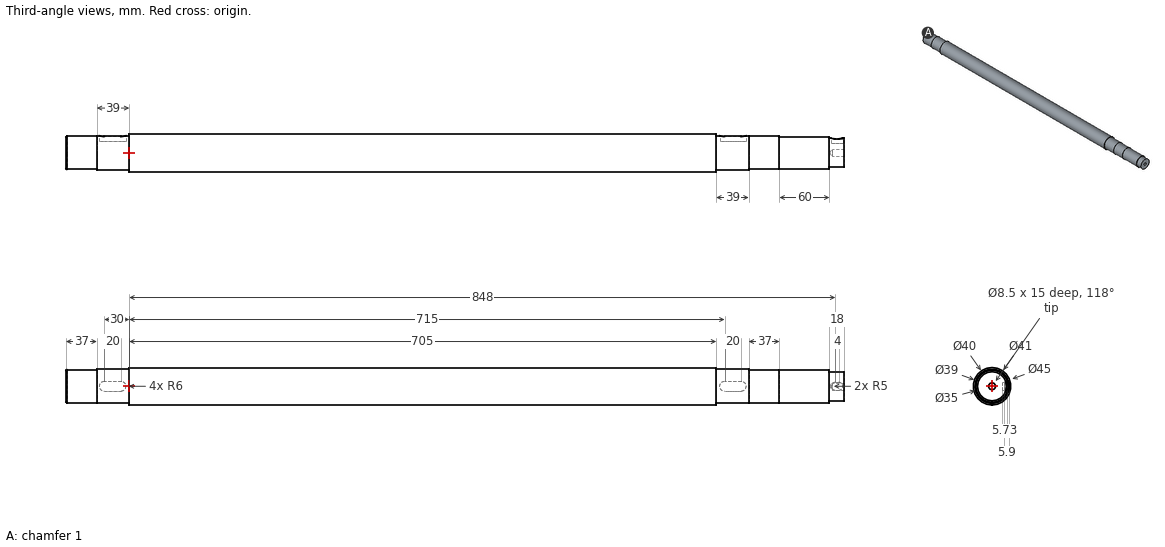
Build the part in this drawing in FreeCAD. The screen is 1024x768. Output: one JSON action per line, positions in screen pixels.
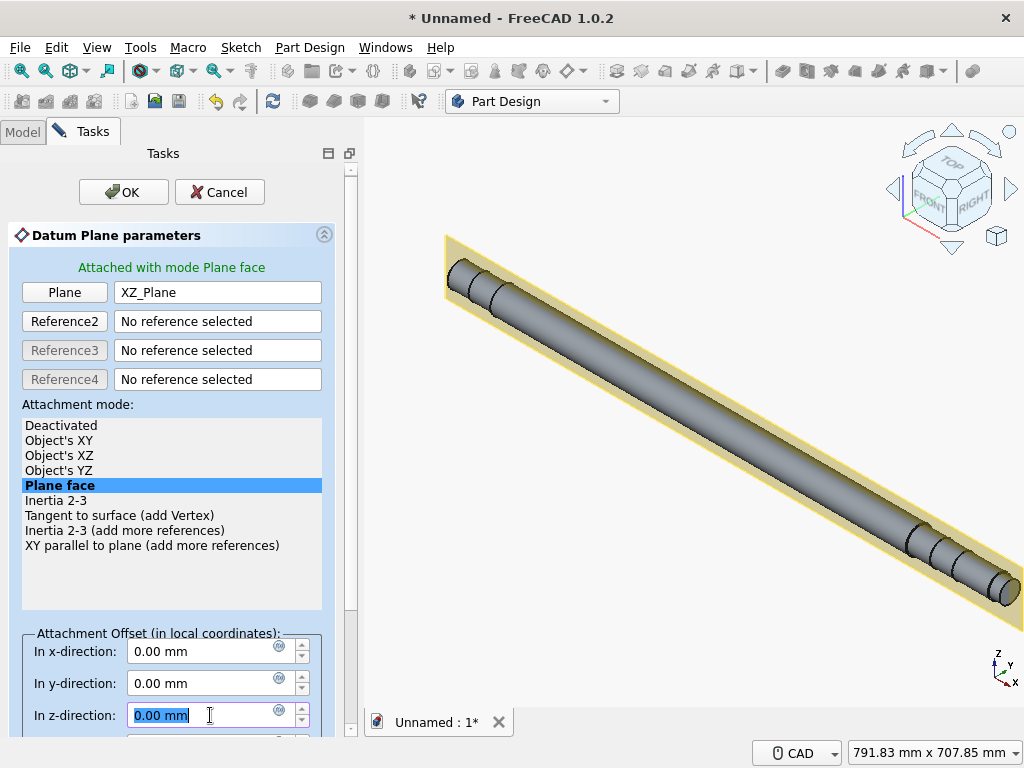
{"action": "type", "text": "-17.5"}
{"action": "key", "text": "Tab"}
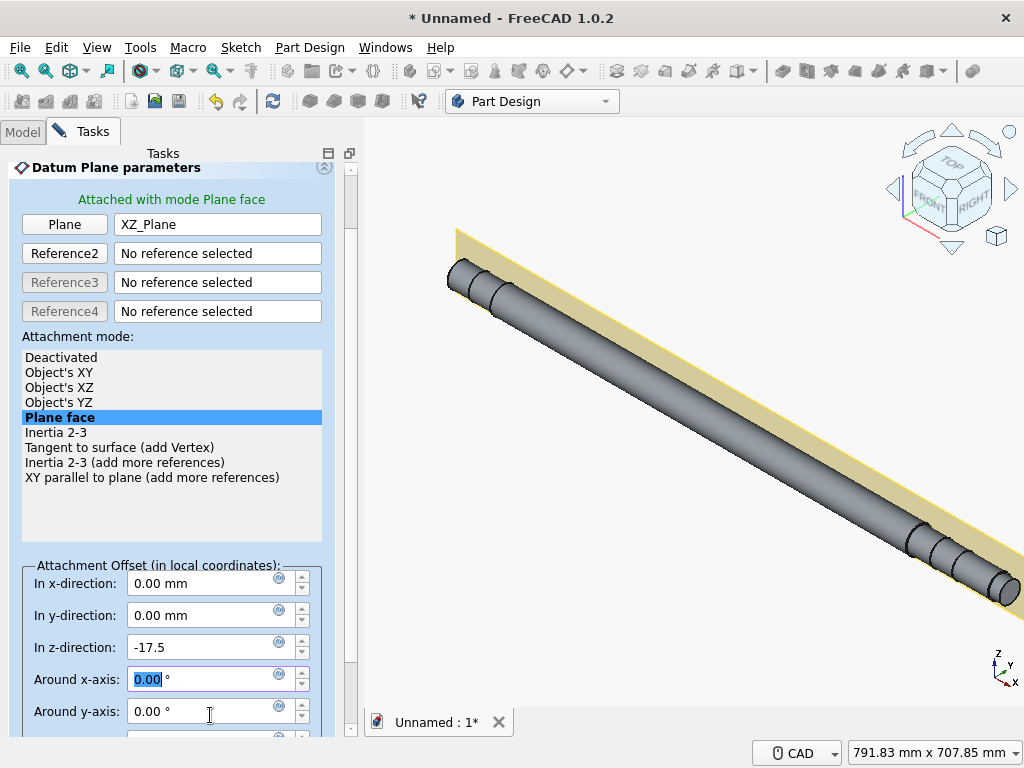
{"action": "scroll", "coordinate": [351, 450], "scroll_direction": "up", "scroll_amount": 2}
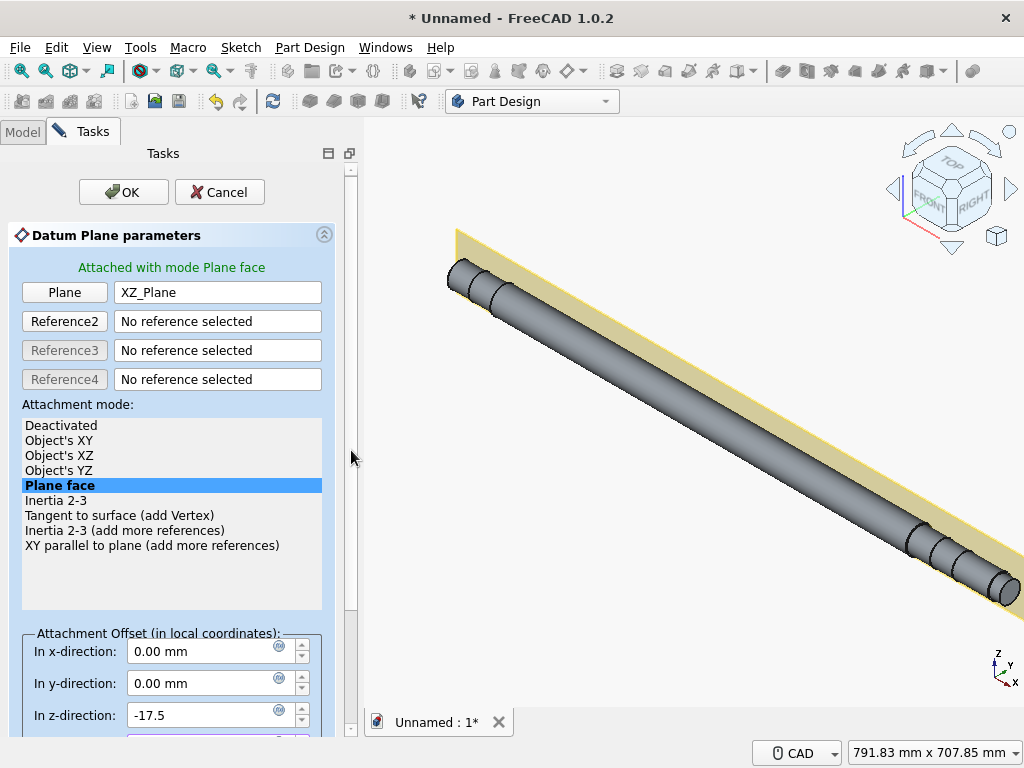
{"action": "left_click", "coordinate": [124, 192]}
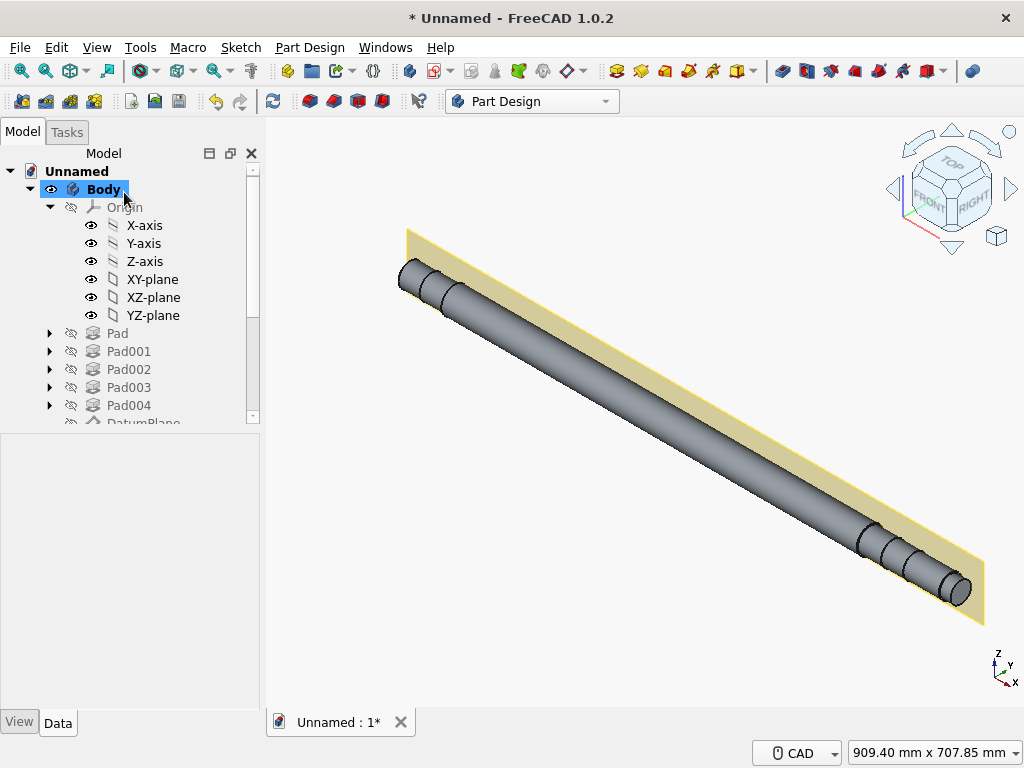
{"action": "scroll", "coordinate": [100, 293], "scroll_direction": "down", "scroll_amount": 3}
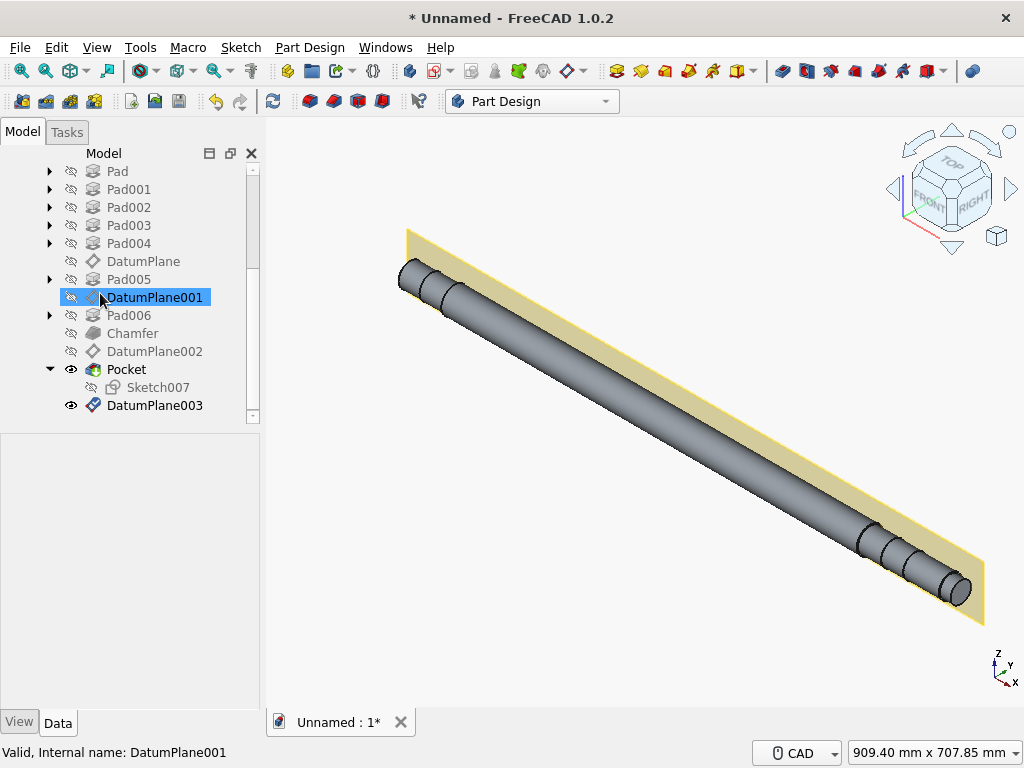
{"action": "left_click", "coordinate": [116, 405]}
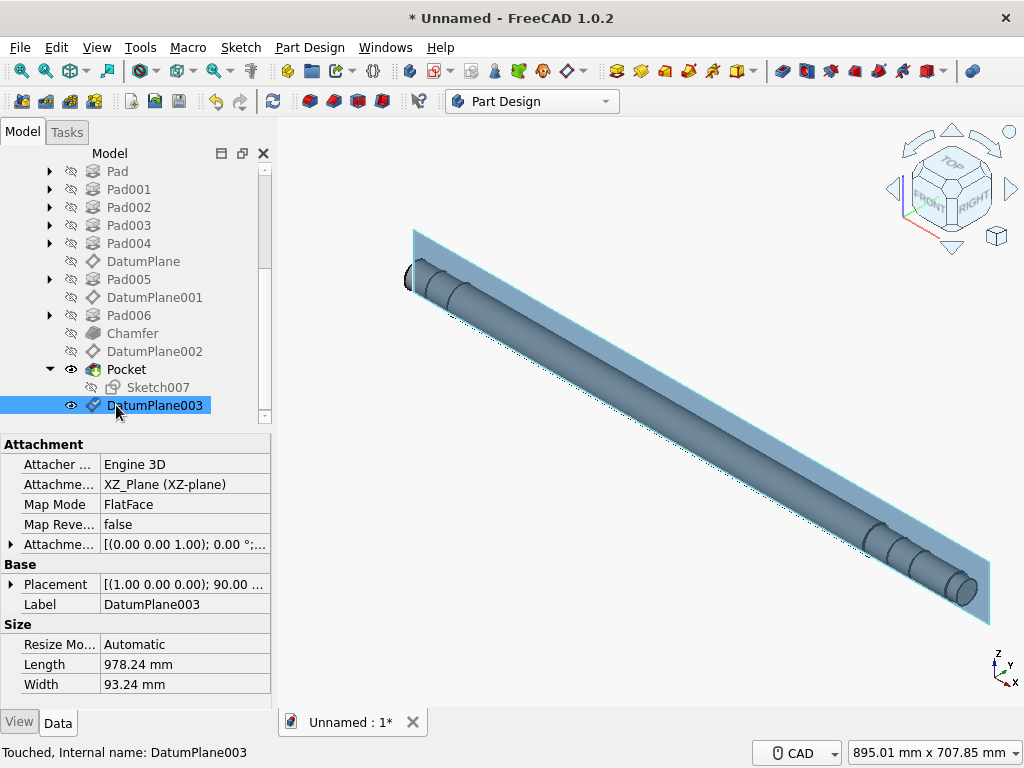
{"action": "left_click", "coordinate": [434, 72]}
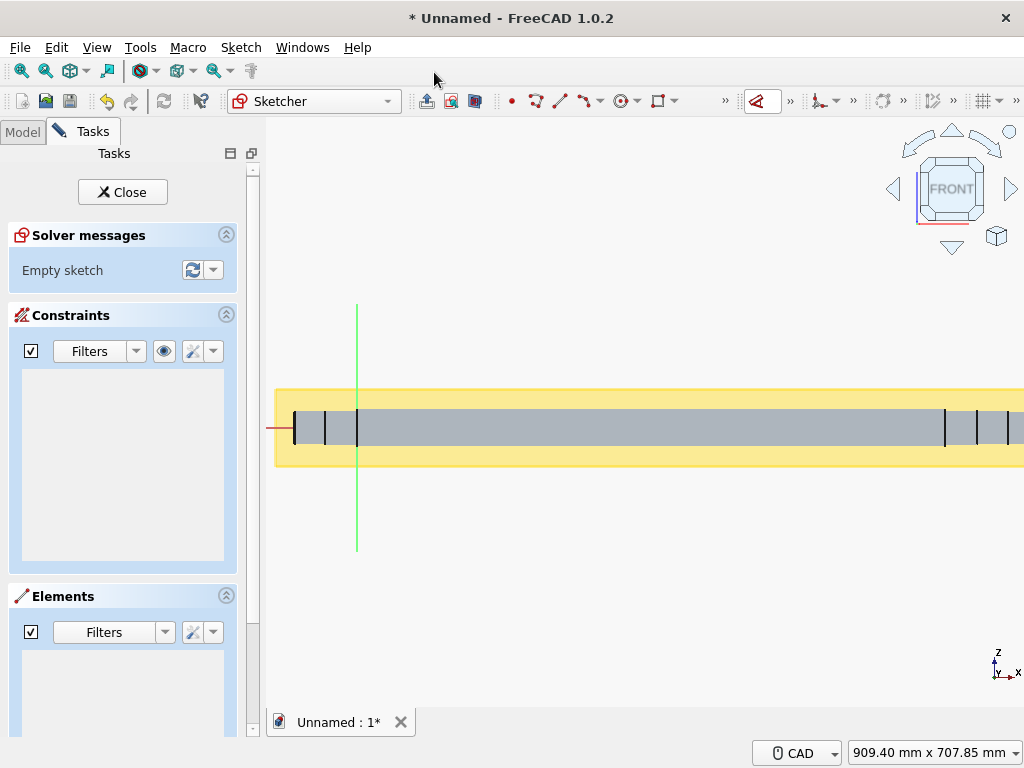
{"action": "left_click", "coordinate": [476, 102]}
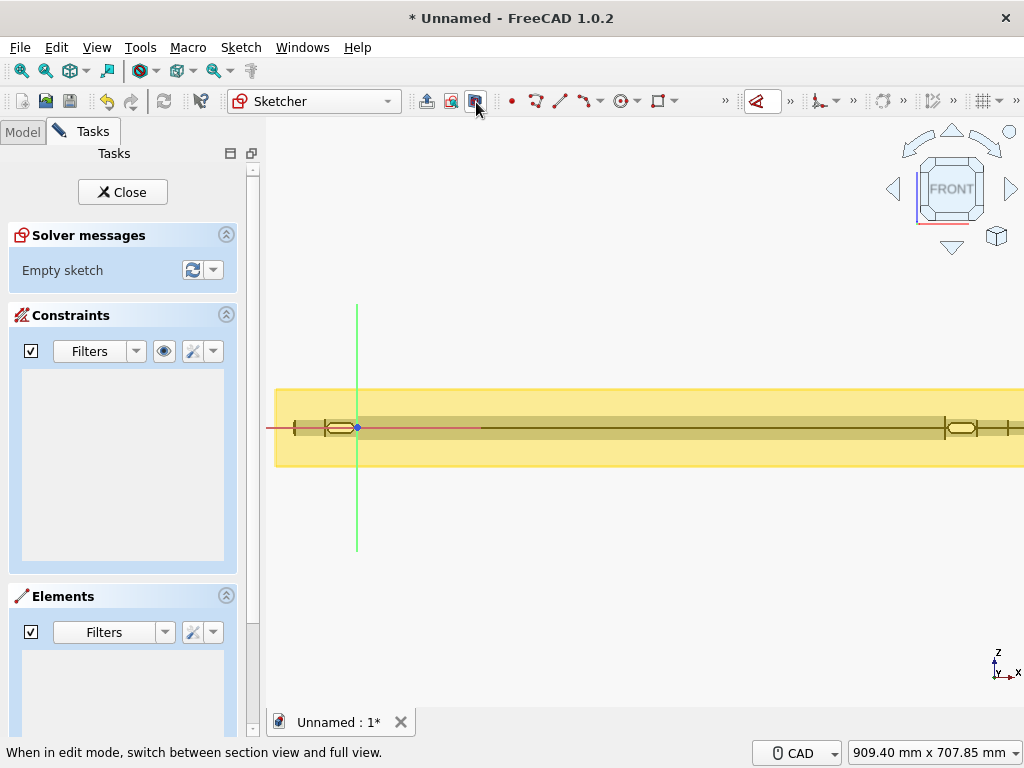
{"action": "scroll", "coordinate": [576, 412], "scroll_direction": "down", "scroll_amount": 5}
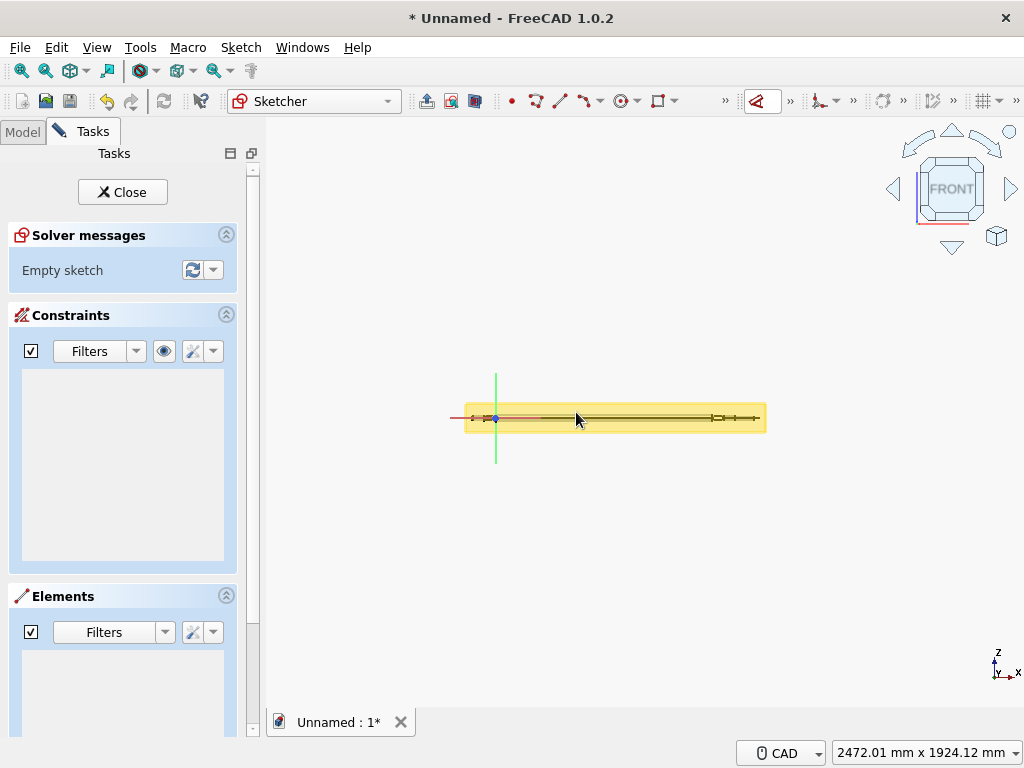
{"action": "scroll", "coordinate": [766, 418], "scroll_direction": "up", "scroll_amount": 15}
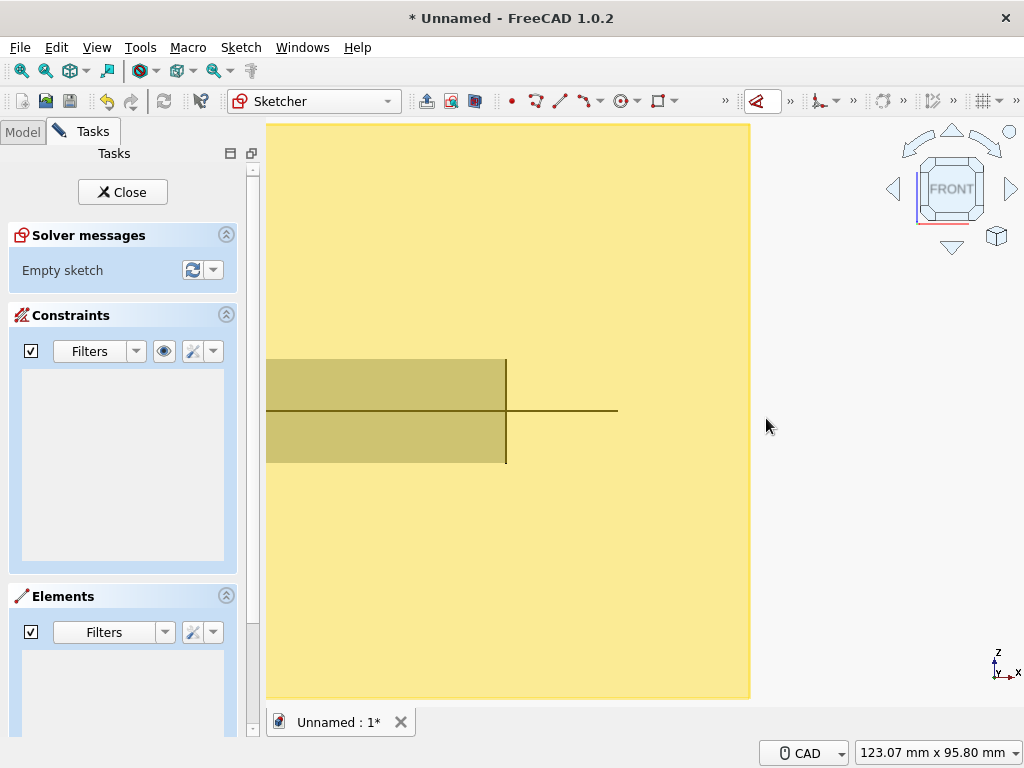
{"action": "scroll", "coordinate": [557, 411], "scroll_direction": "up", "scroll_amount": 8}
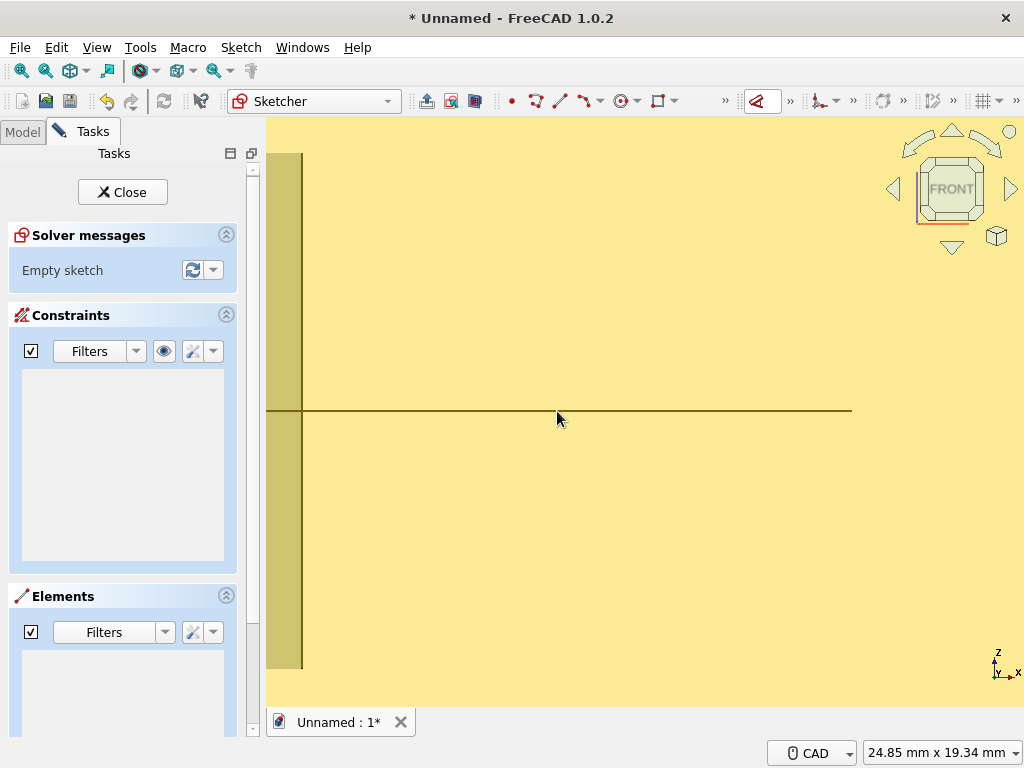
{"action": "key", "text": "g s"}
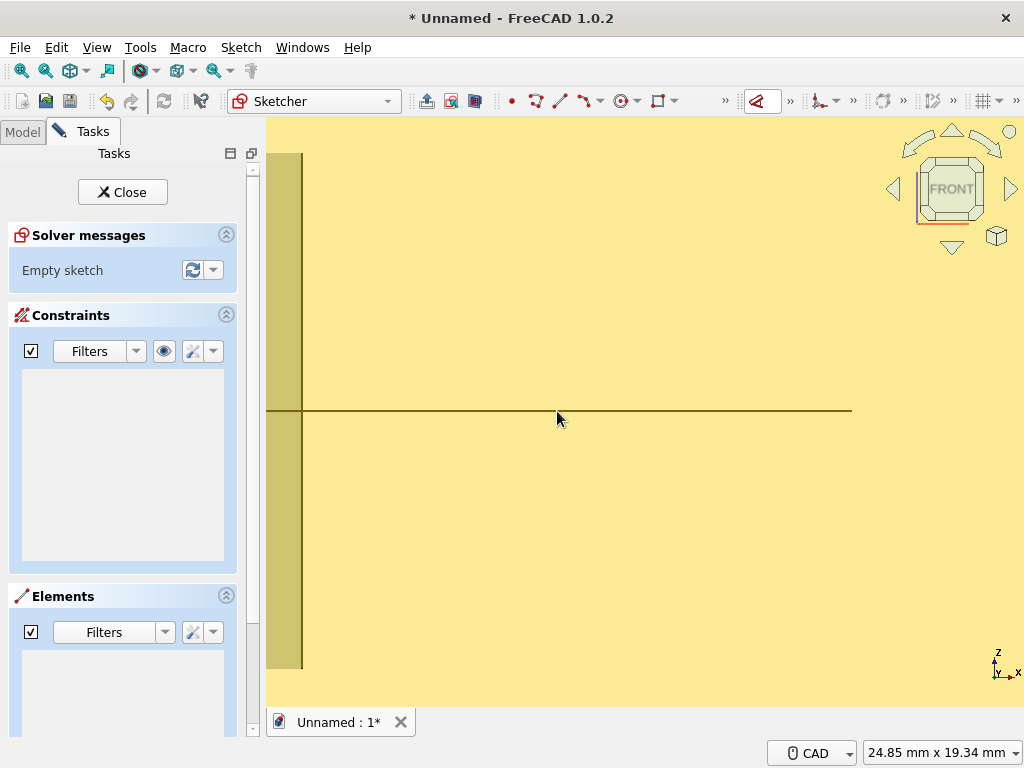
{"action": "left_click", "coordinate": [516, 411]}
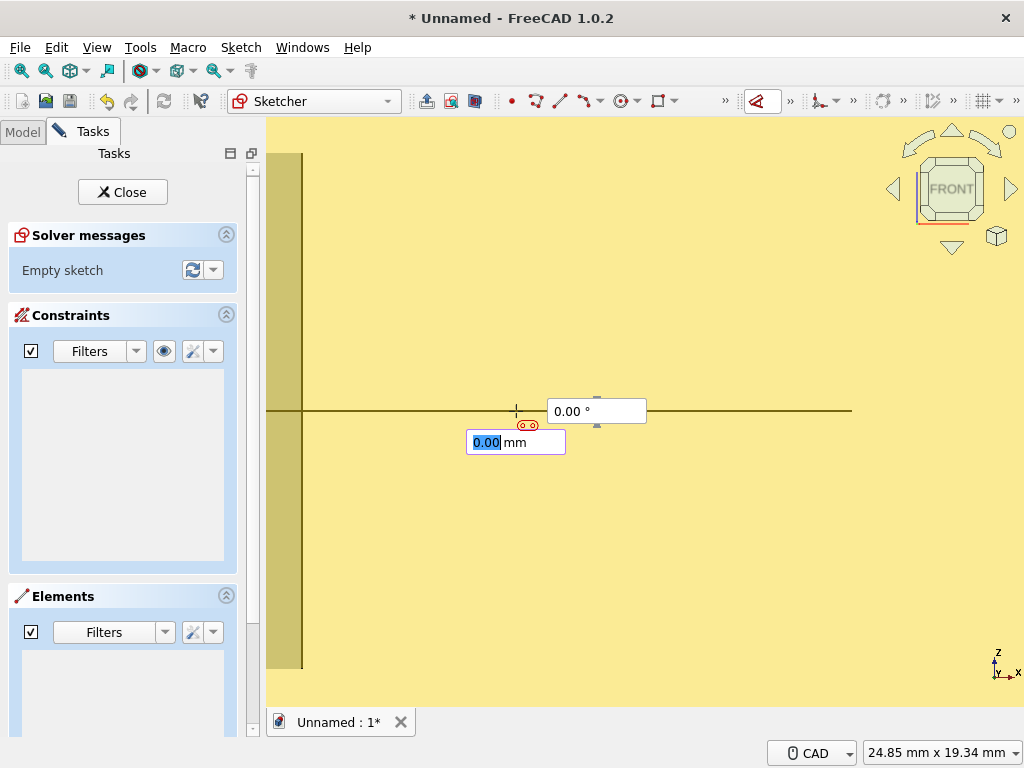
{"action": "left_click", "coordinate": [638, 402]}